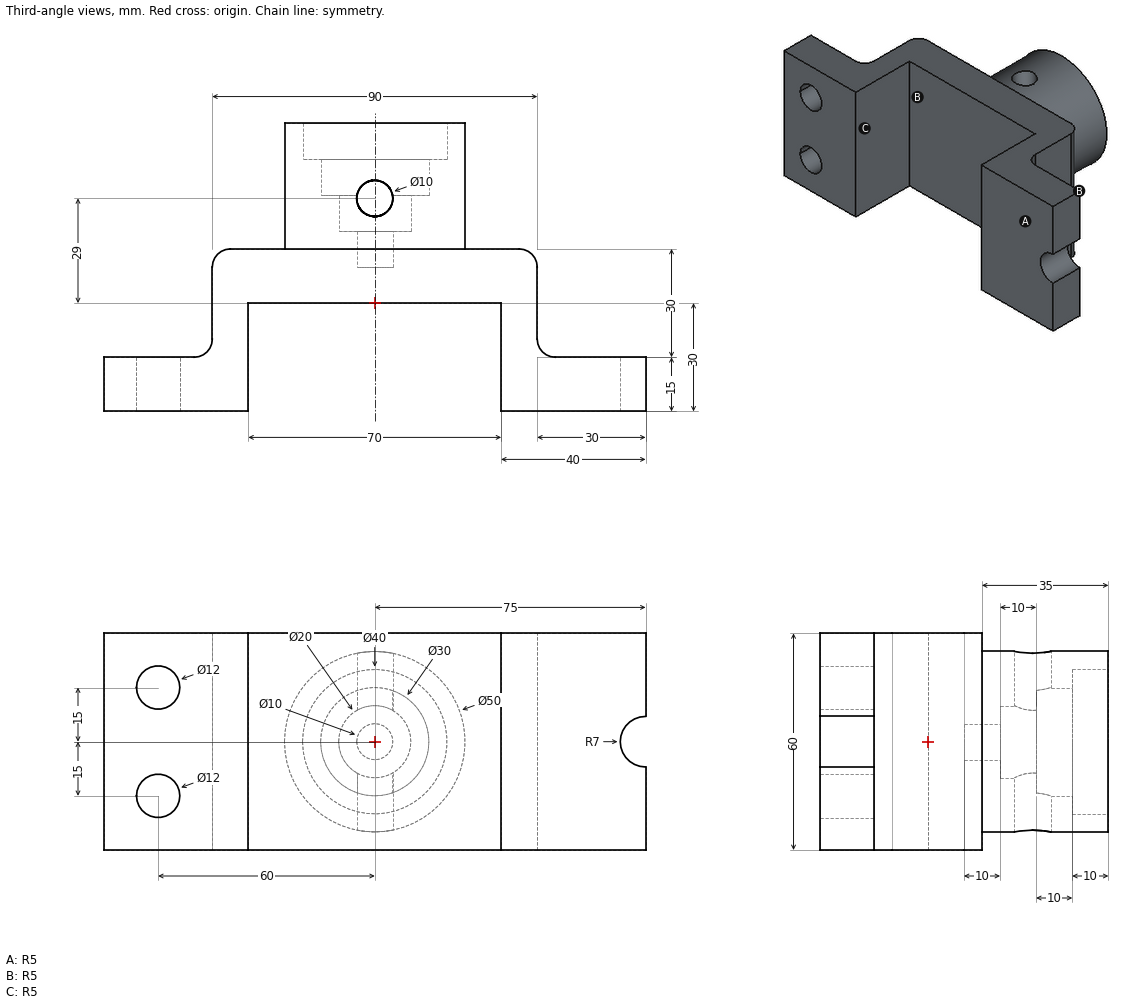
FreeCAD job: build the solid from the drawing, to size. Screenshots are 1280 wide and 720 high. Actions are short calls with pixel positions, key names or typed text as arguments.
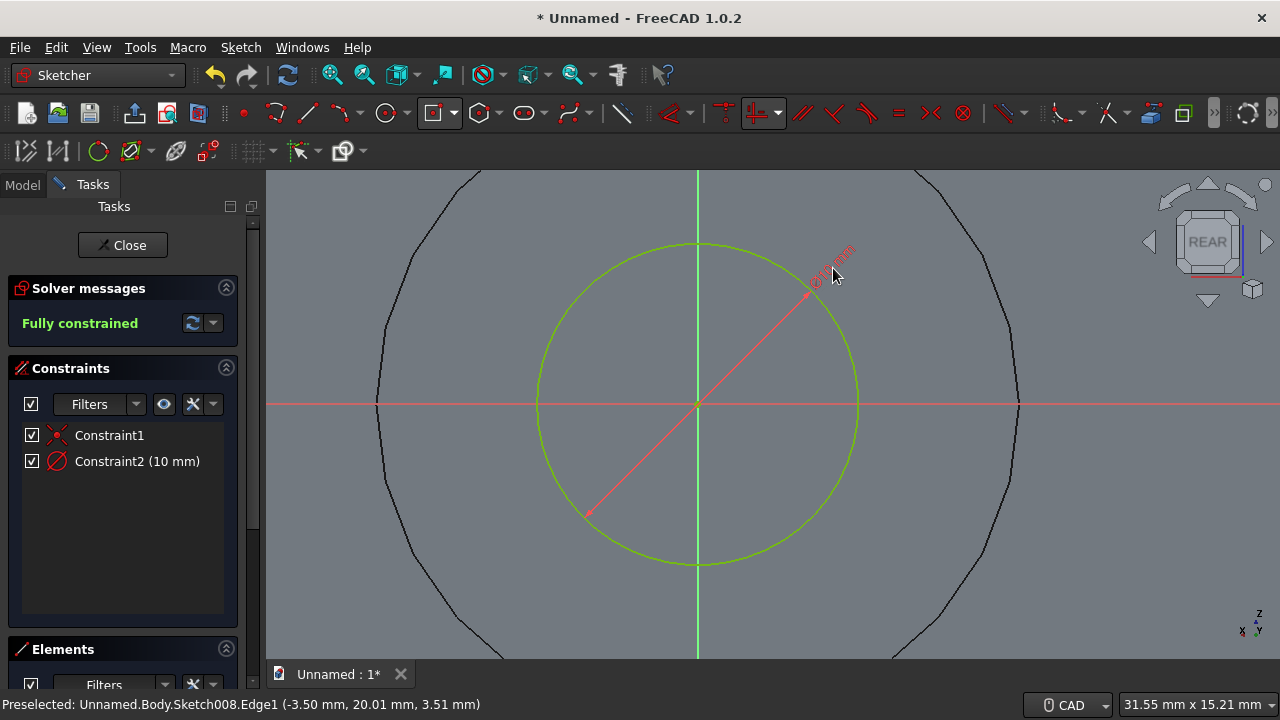
click(123, 245)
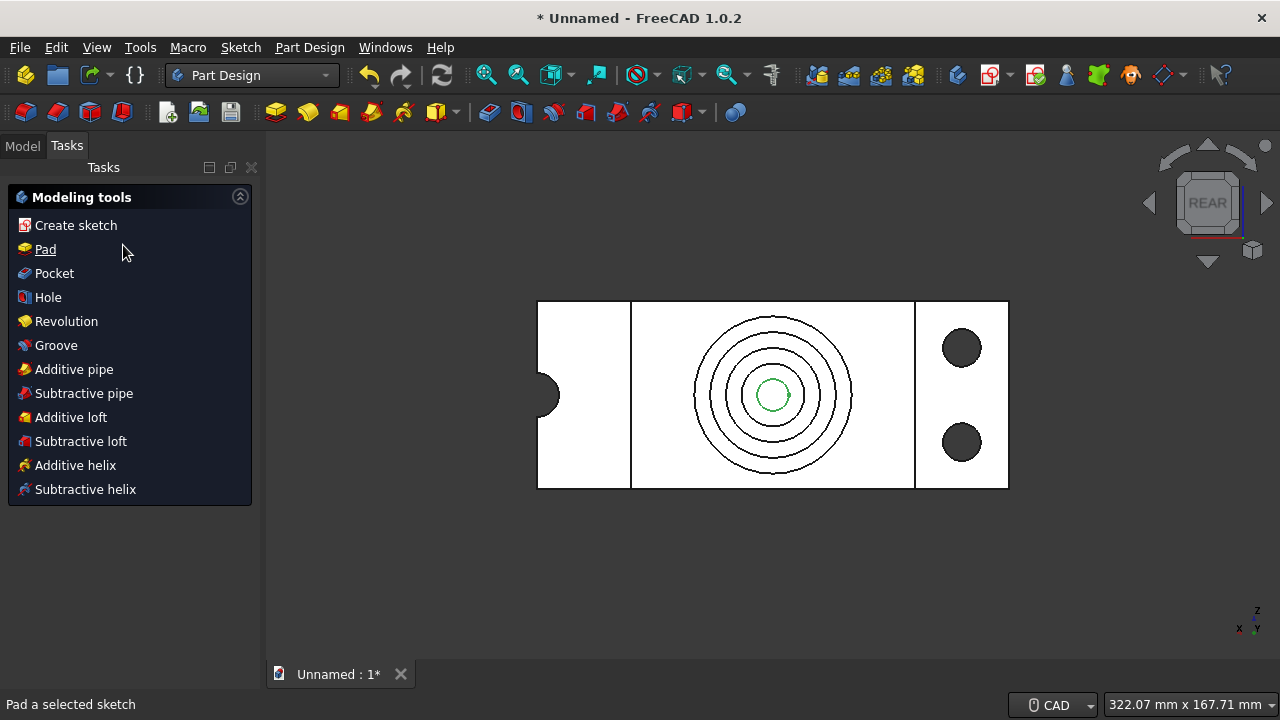
click(490, 112)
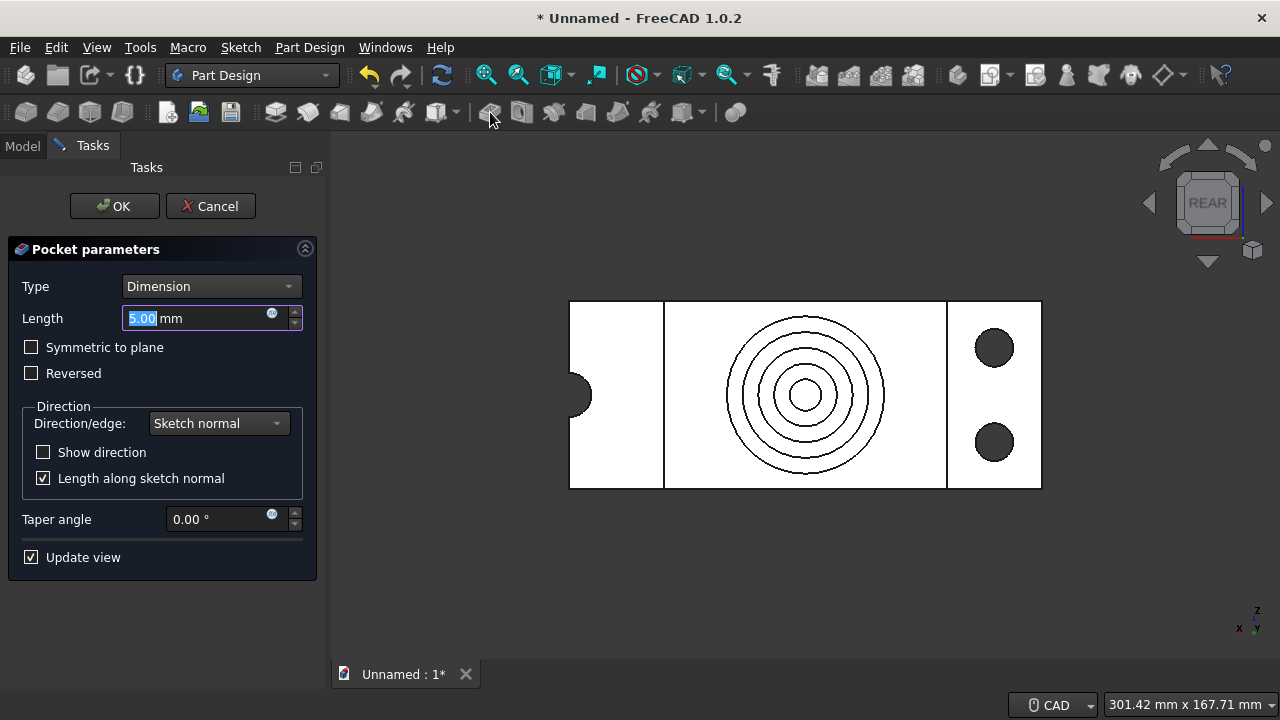
text(10)
key(Tab)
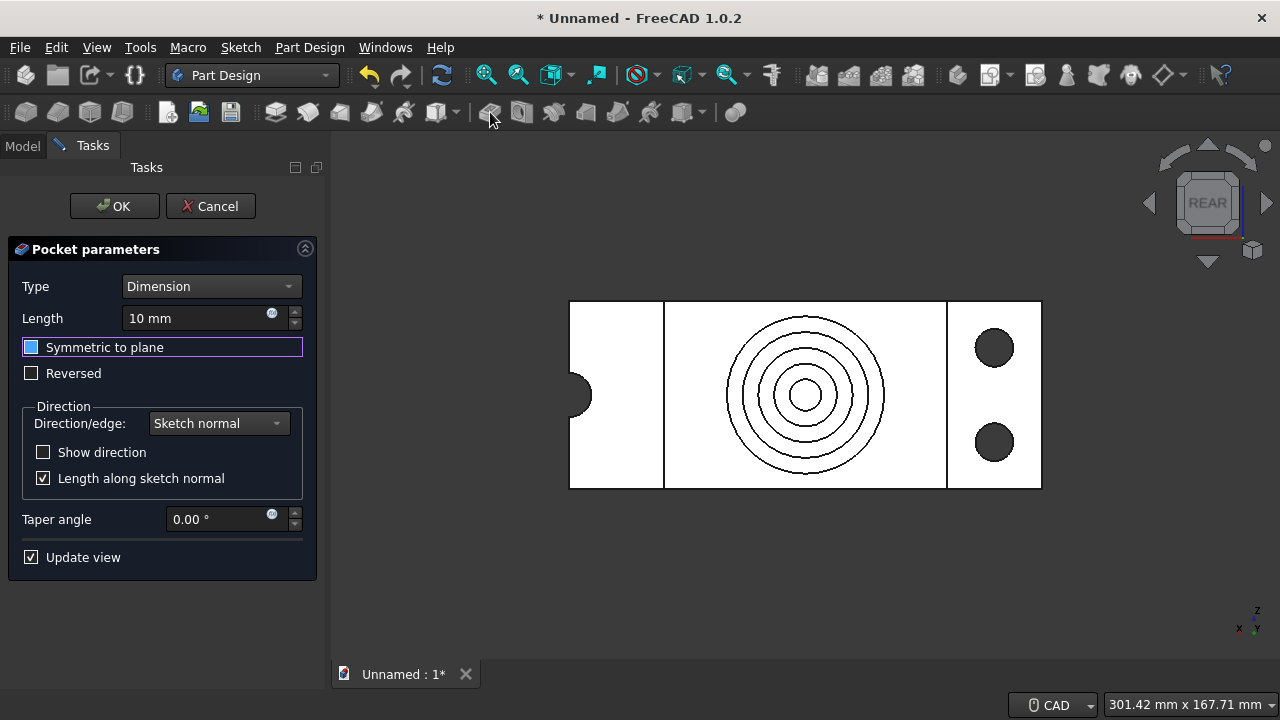
click(115, 206)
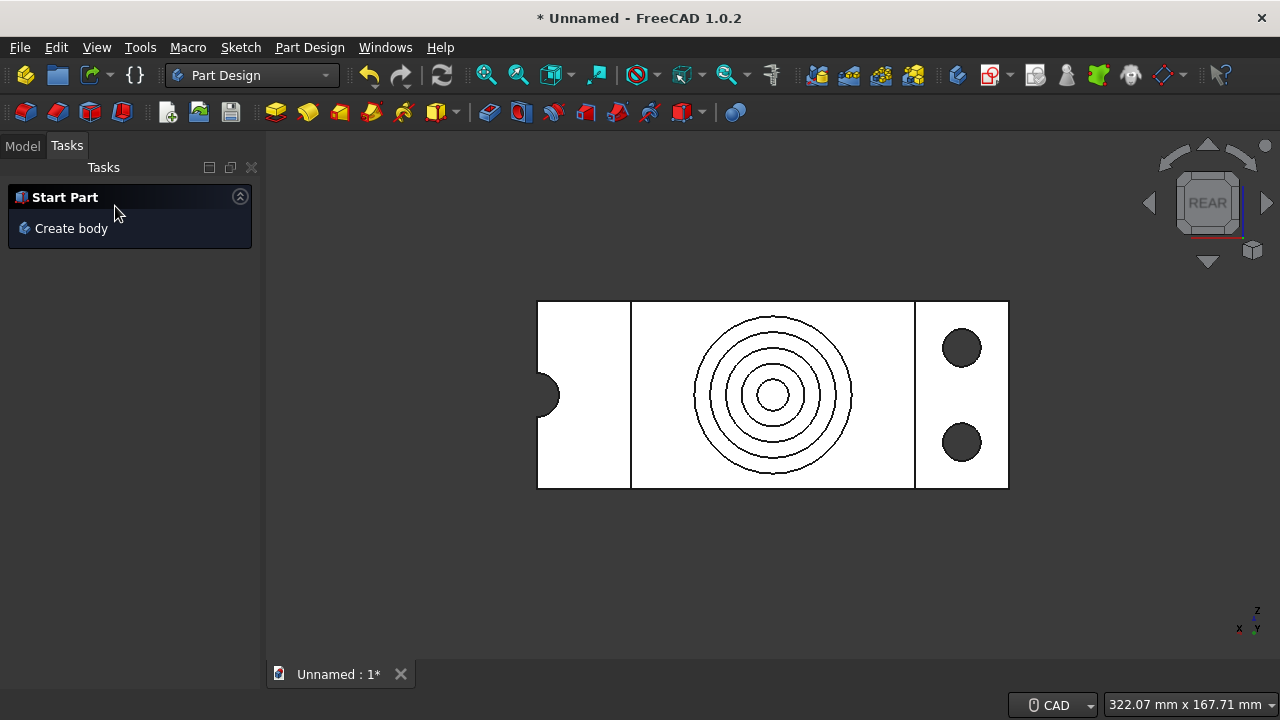
key(0)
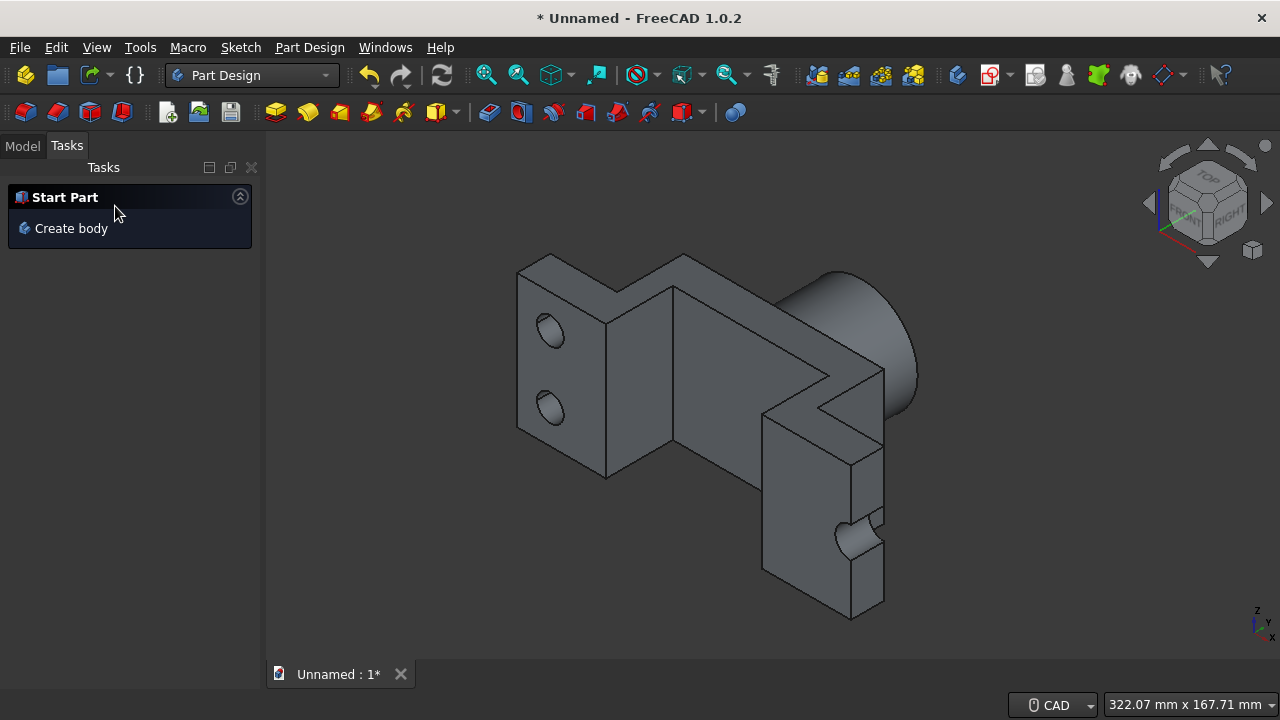
click(610, 301)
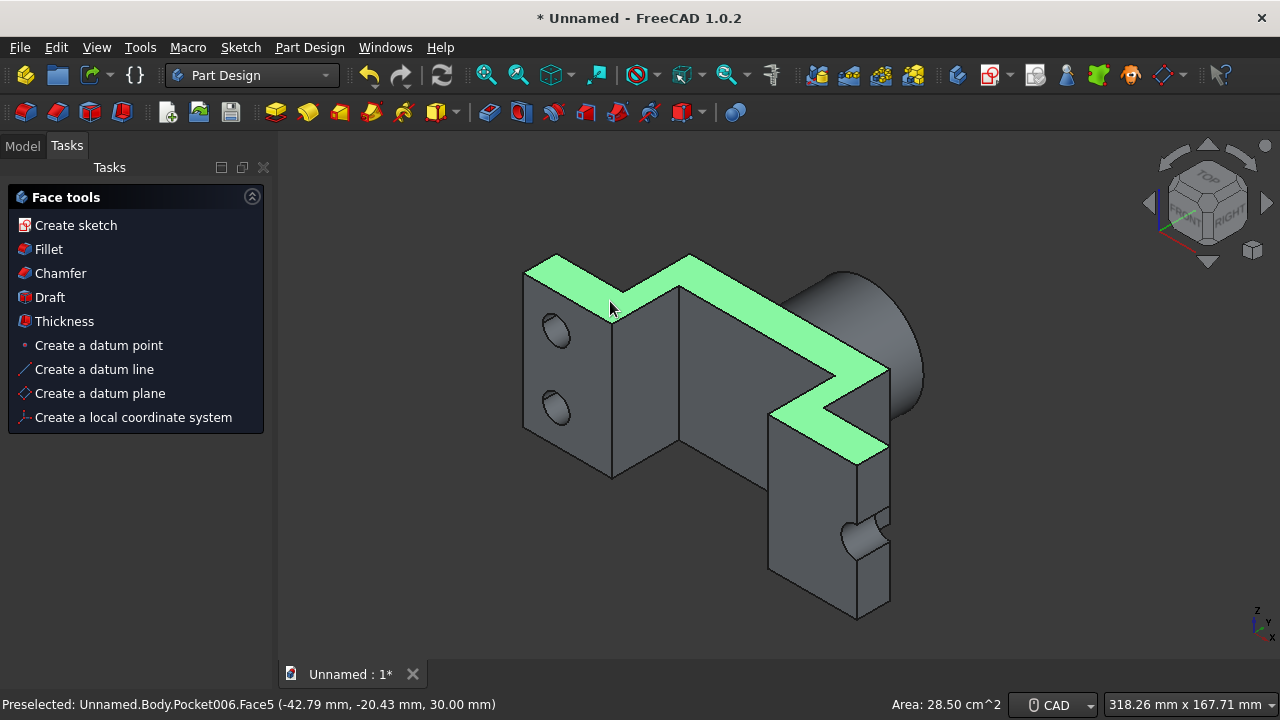
click(990, 76)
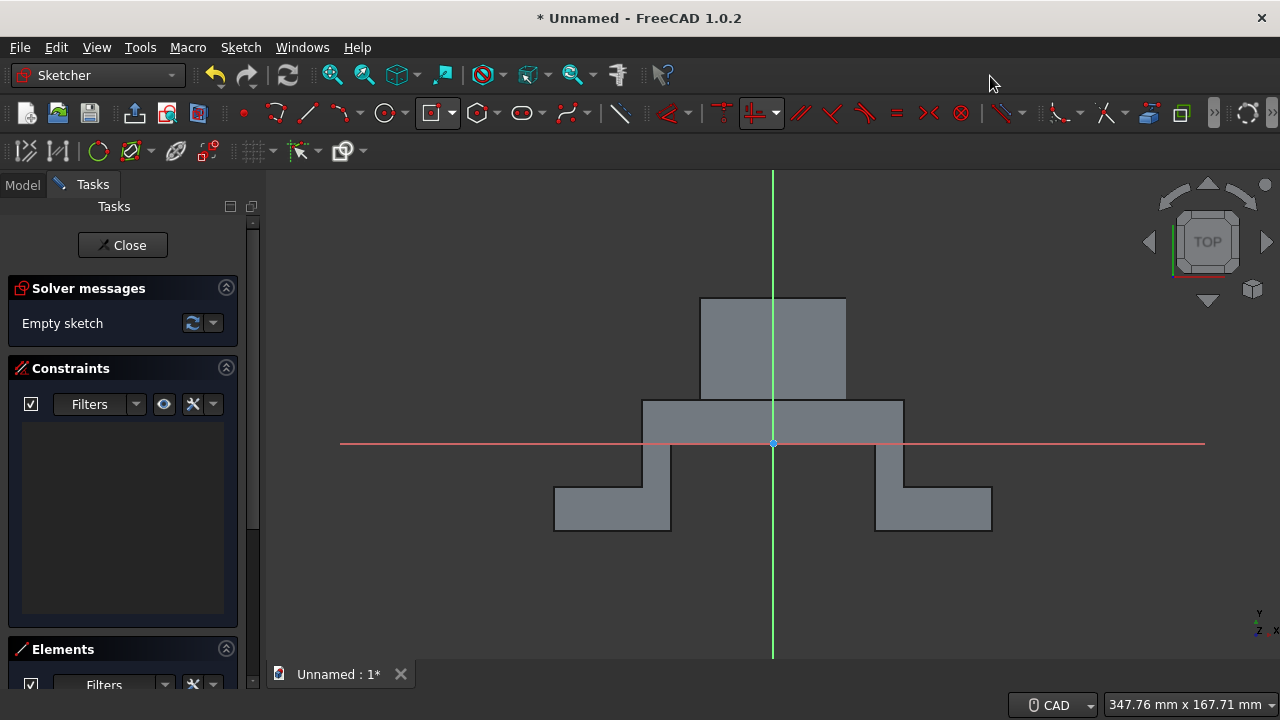
scroll(780, 354, up, 12)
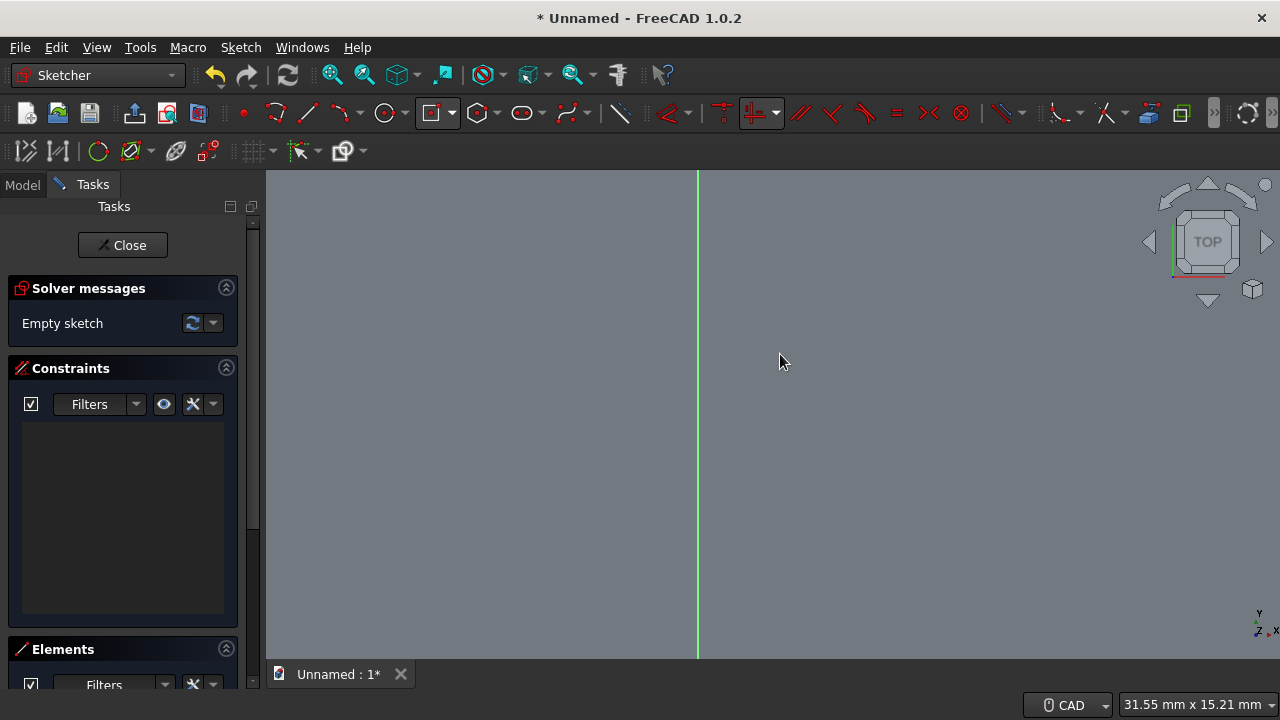
click(386, 114)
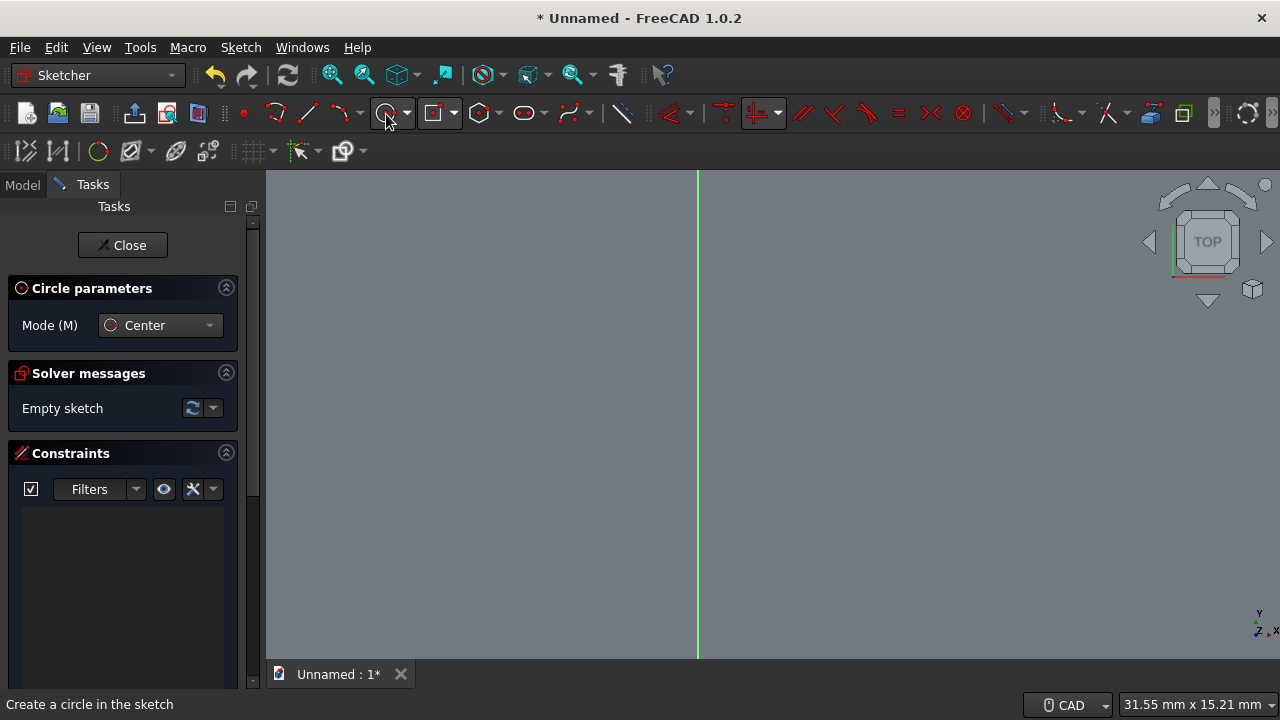
click(698, 406)
click(811, 293)
key(Escape)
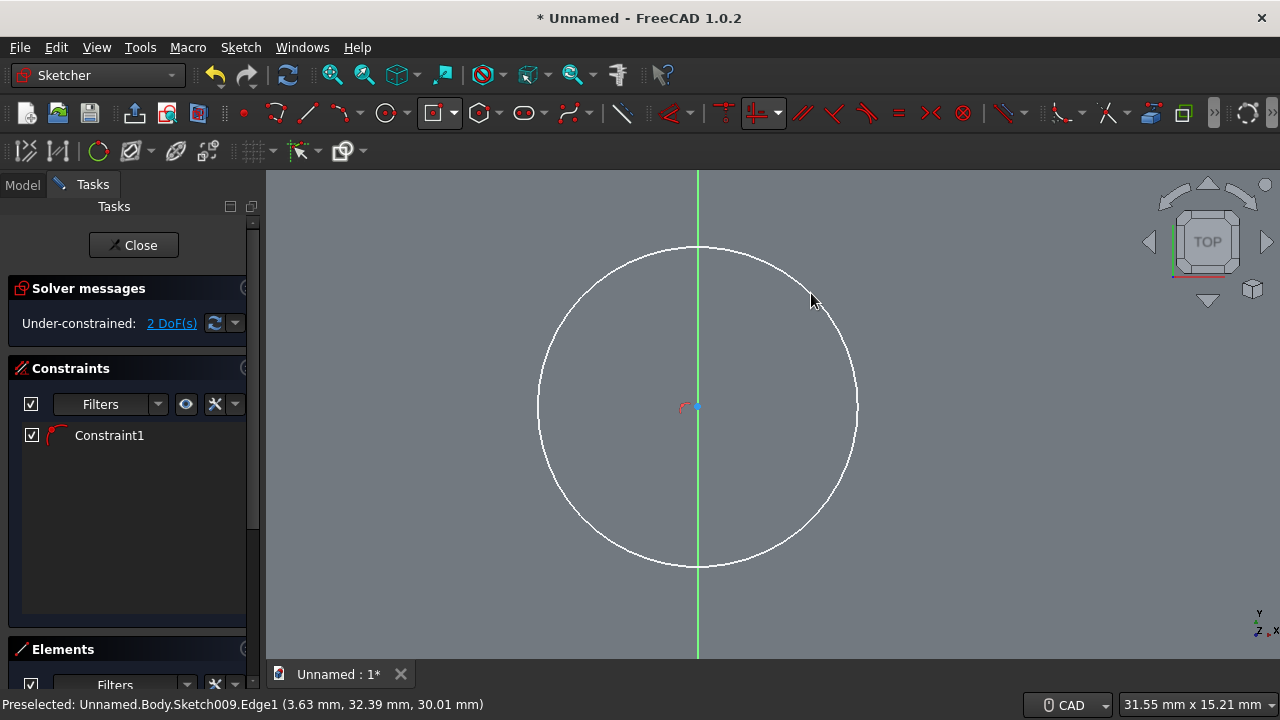
click(670, 114)